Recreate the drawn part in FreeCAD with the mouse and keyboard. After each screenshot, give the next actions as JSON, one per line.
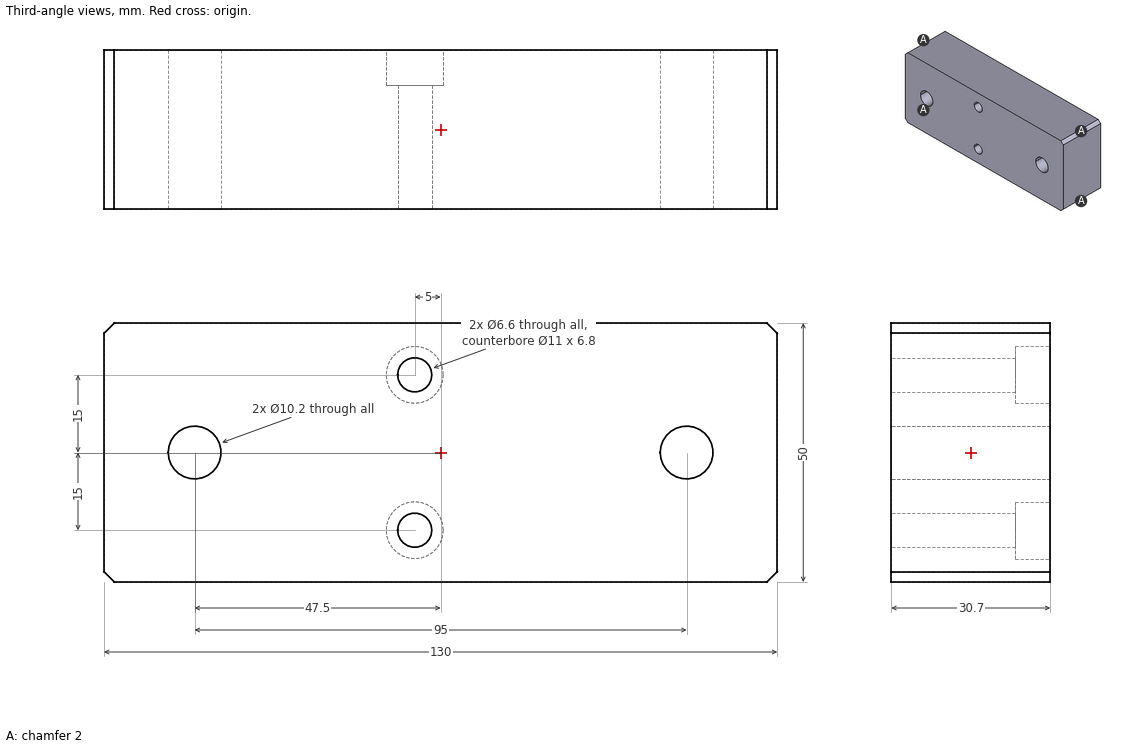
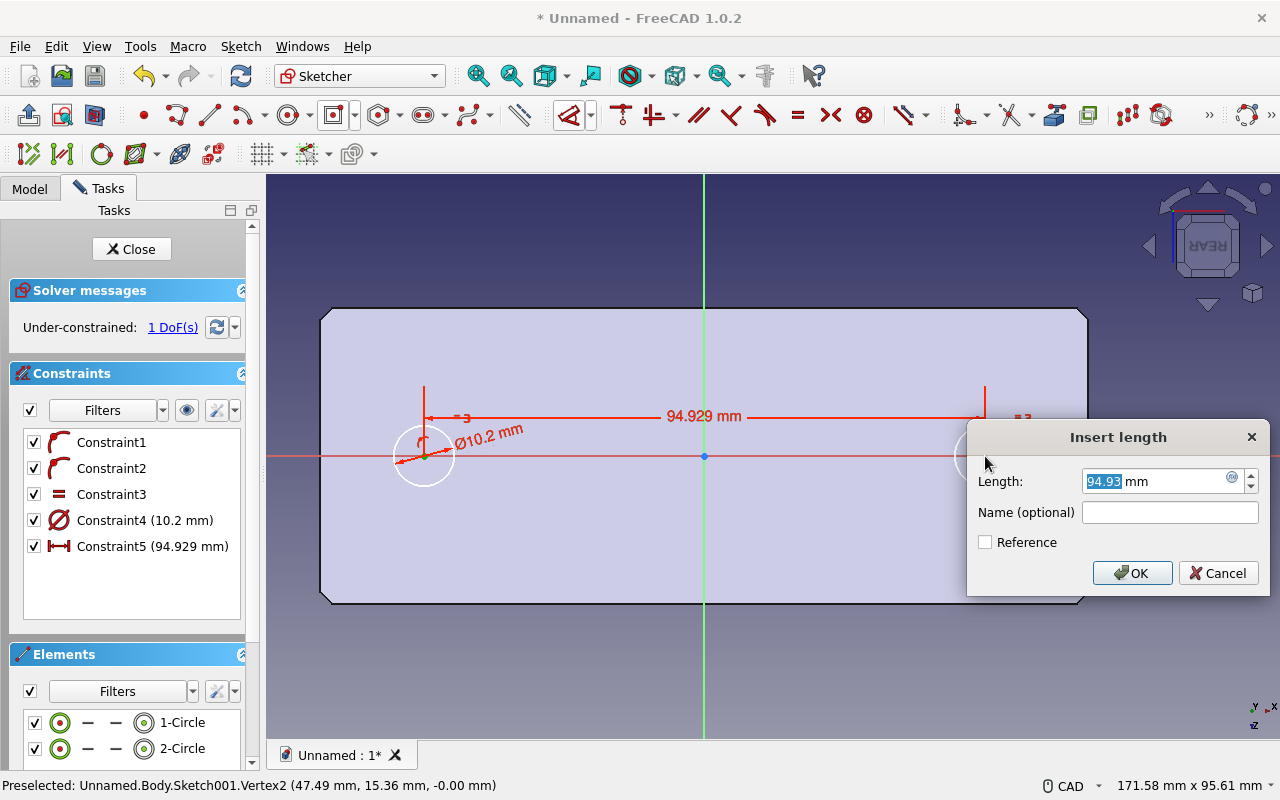
{"action": "type", "text": "95"}
{"action": "key", "text": "Return"}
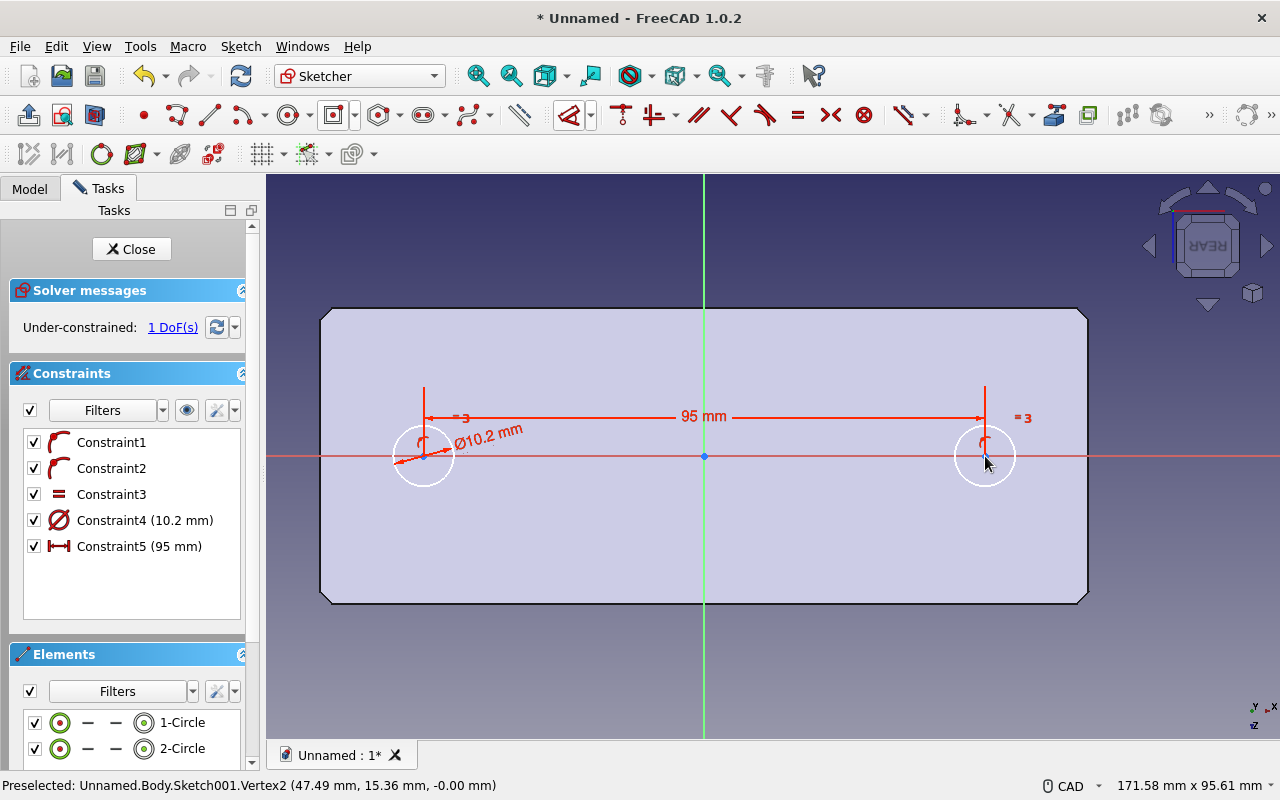
{"action": "left_click", "coordinate": [424, 456]}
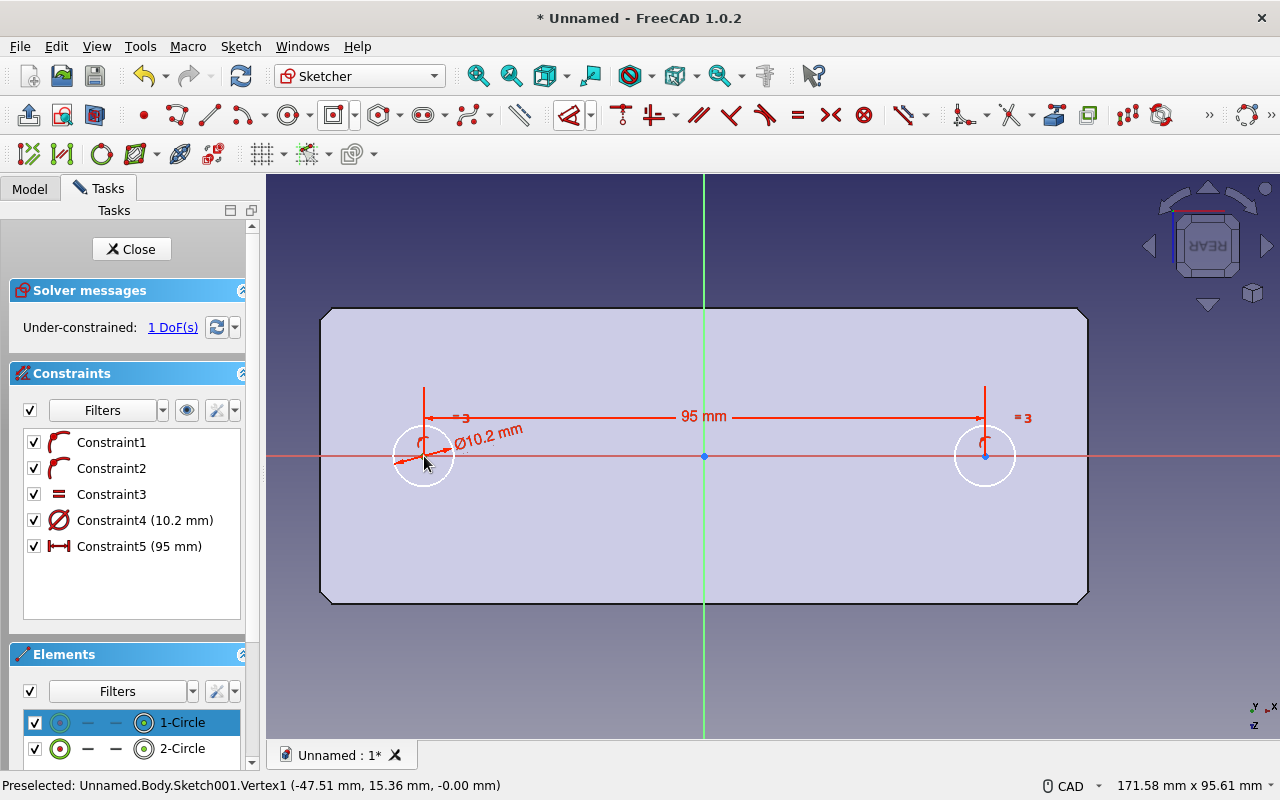
{"action": "key", "text": "l"}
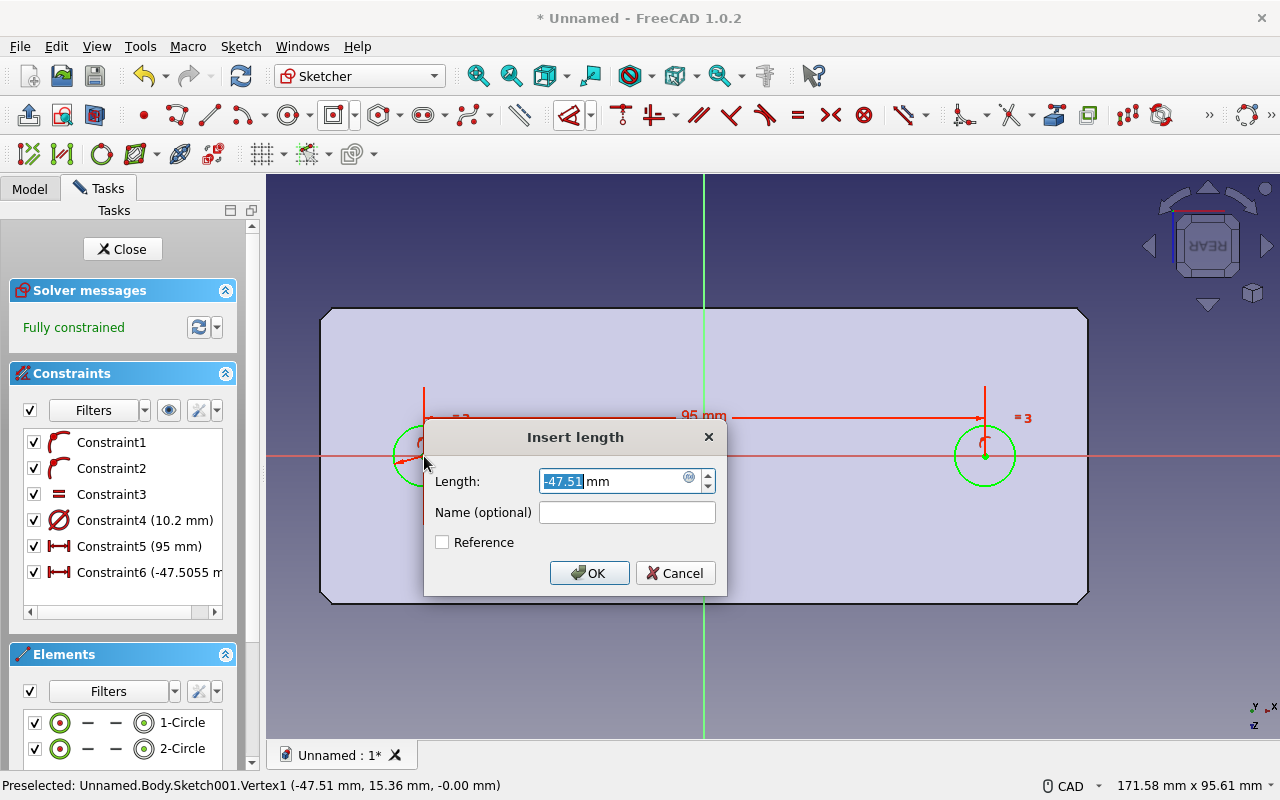
{"action": "type", "text": "-47.5"}
{"action": "key", "text": "Return"}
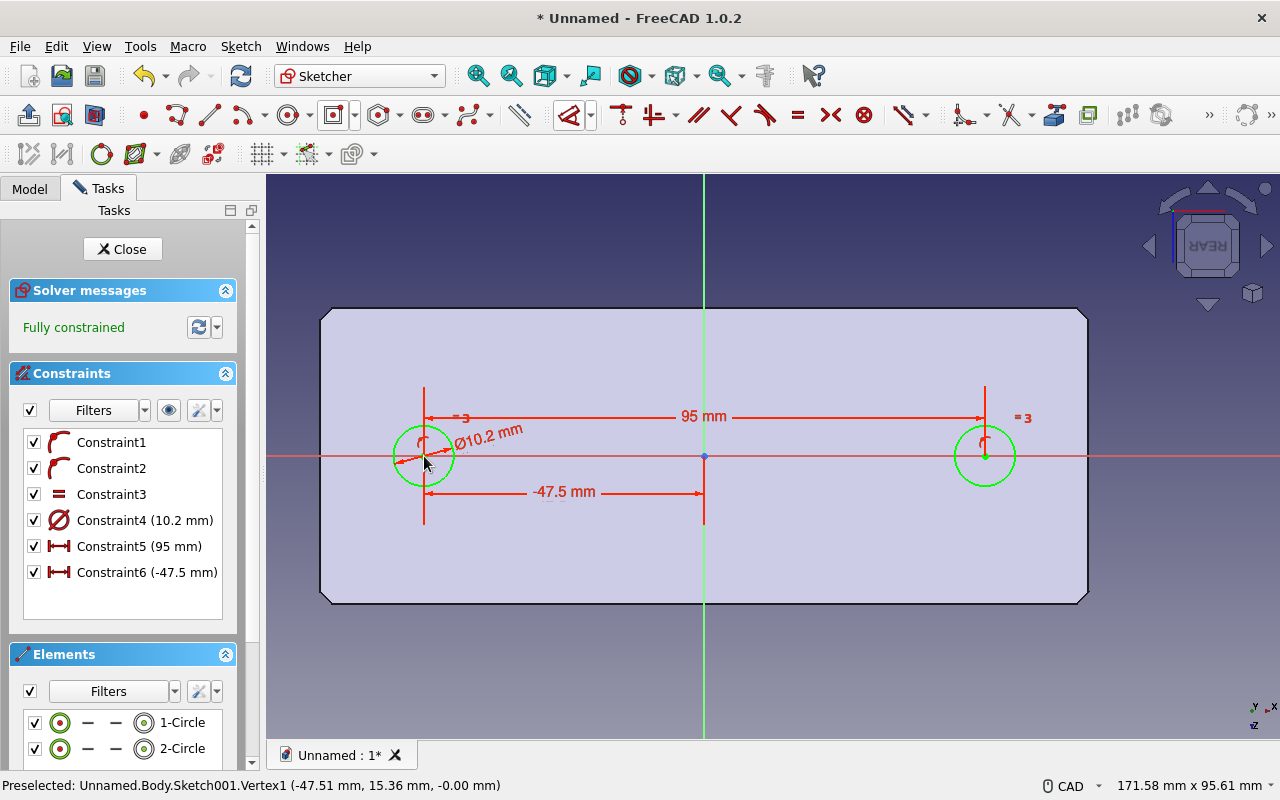
{"action": "left_click", "coordinate": [123, 249]}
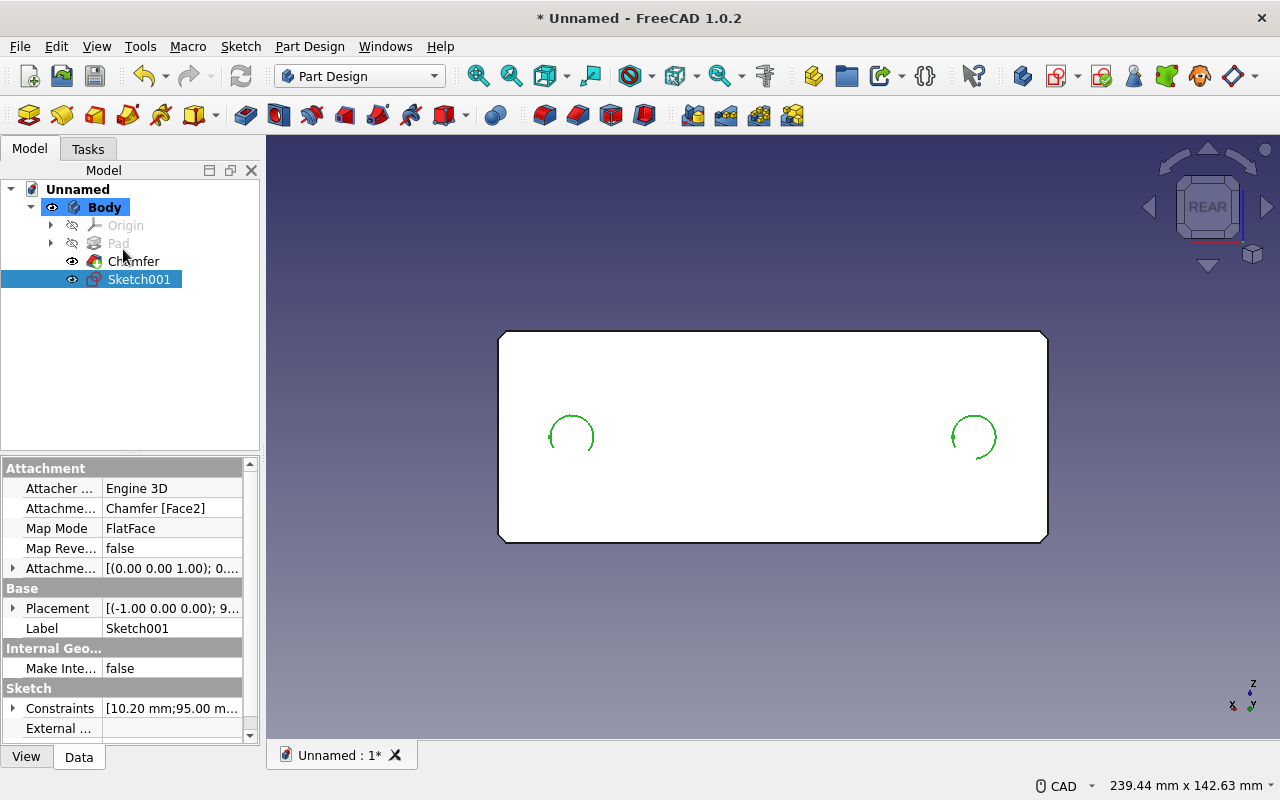
{"action": "left_click", "coordinate": [279, 116]}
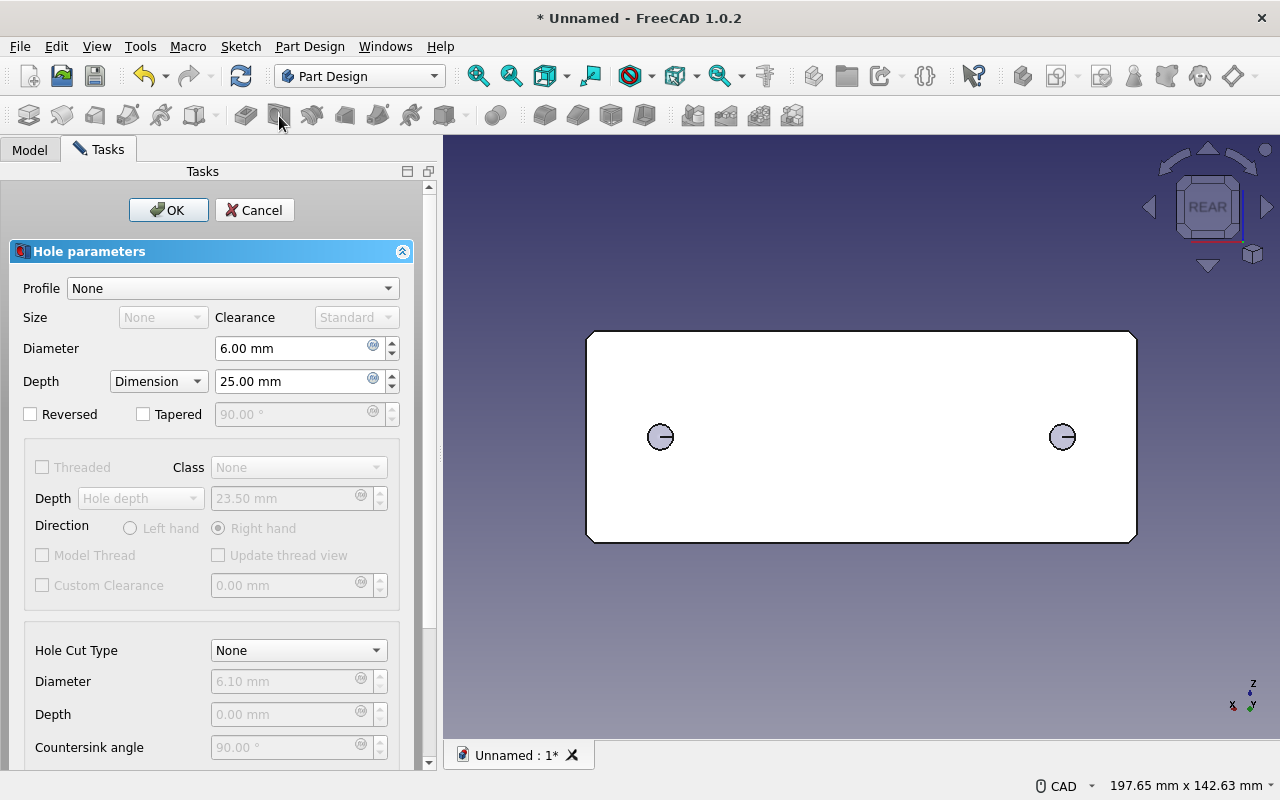
{"action": "triple_click", "coordinate": [300, 348]}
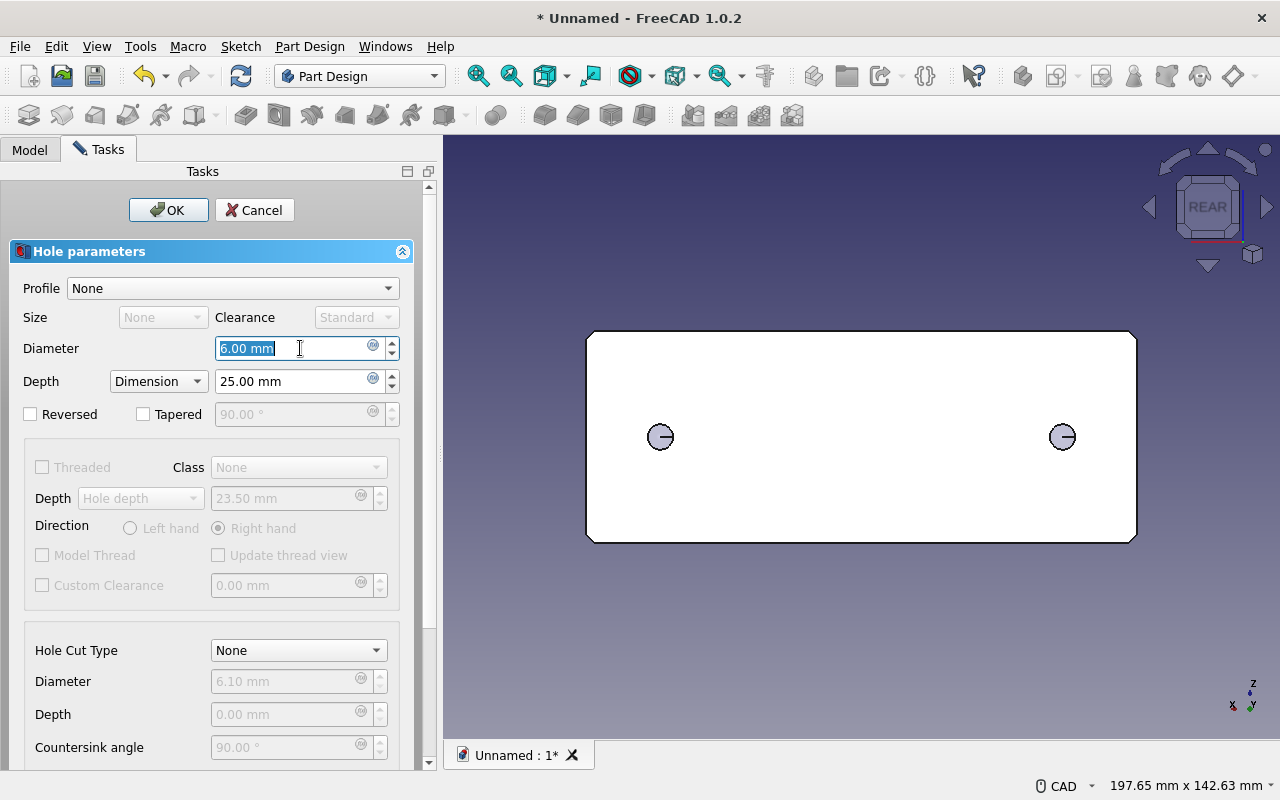
{"action": "type", "text": "10.2"}
{"action": "key", "text": "Tab"}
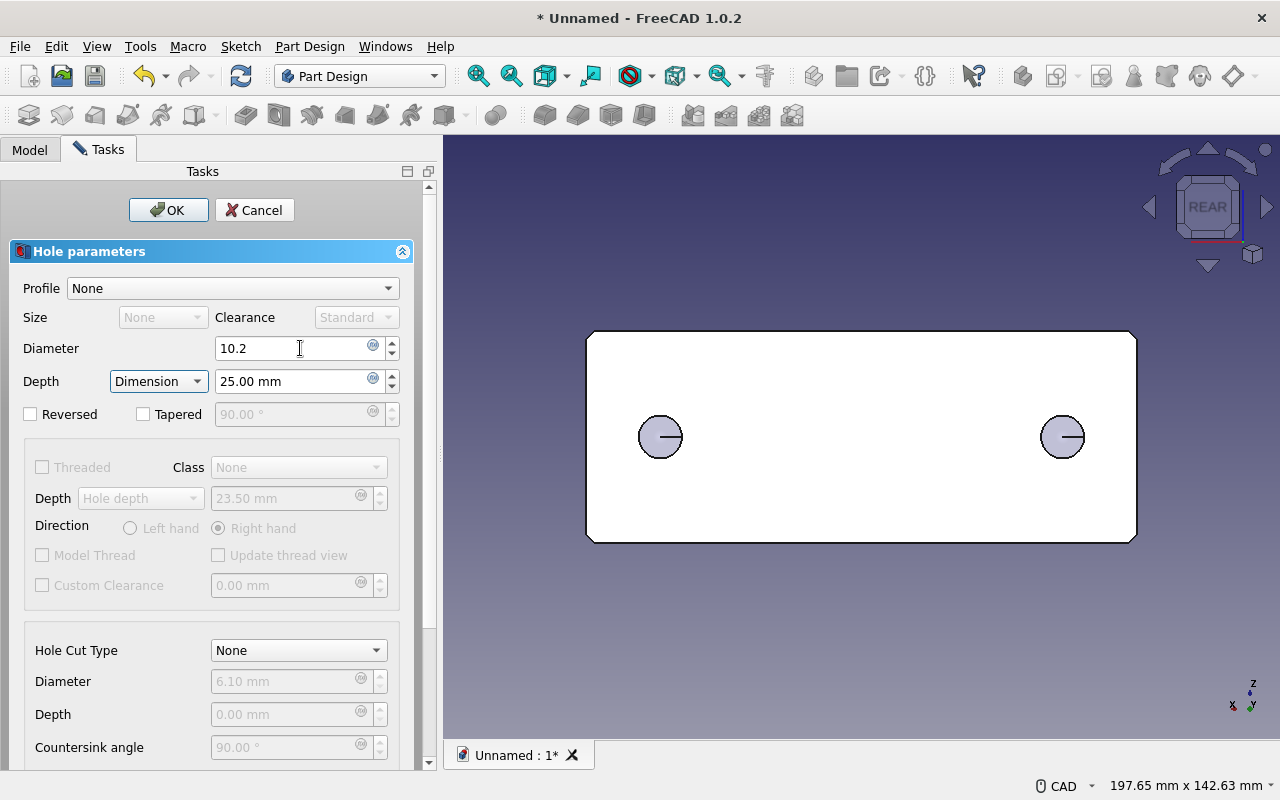
{"action": "left_click", "coordinate": [160, 382]}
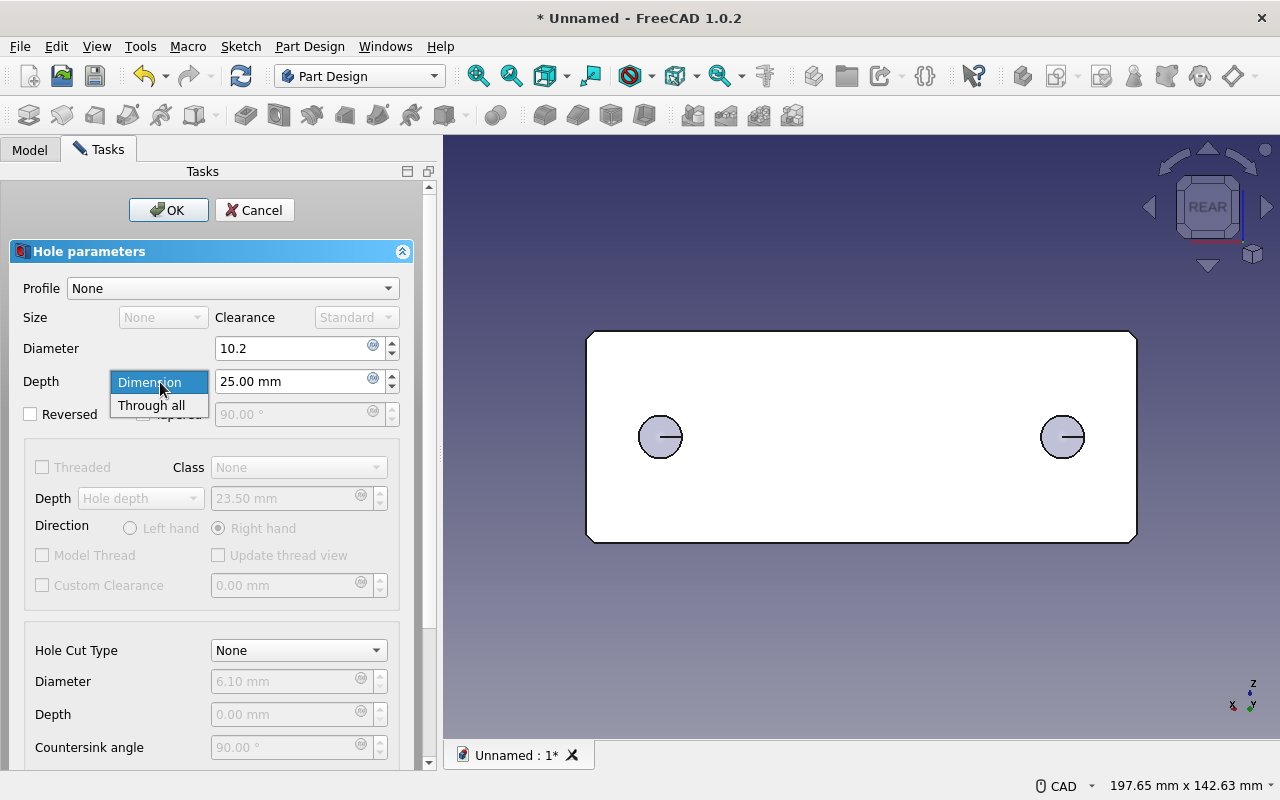
{"action": "left_click", "coordinate": [158, 406]}